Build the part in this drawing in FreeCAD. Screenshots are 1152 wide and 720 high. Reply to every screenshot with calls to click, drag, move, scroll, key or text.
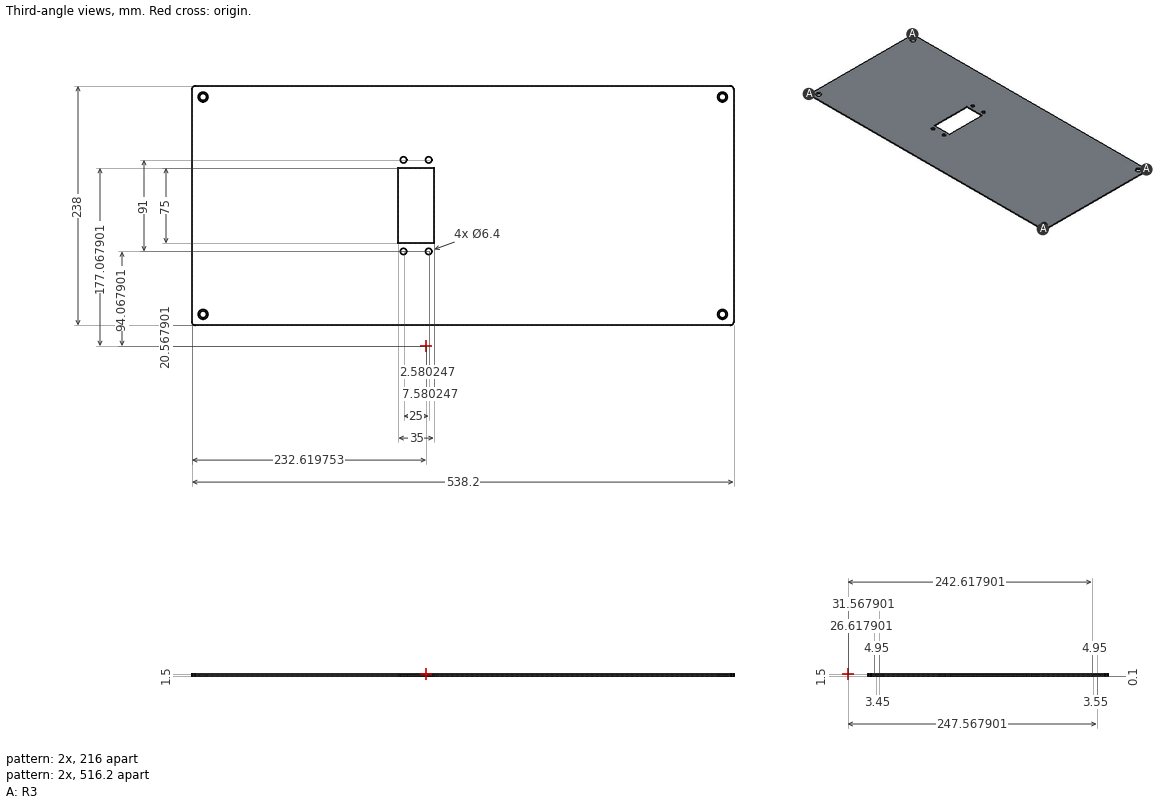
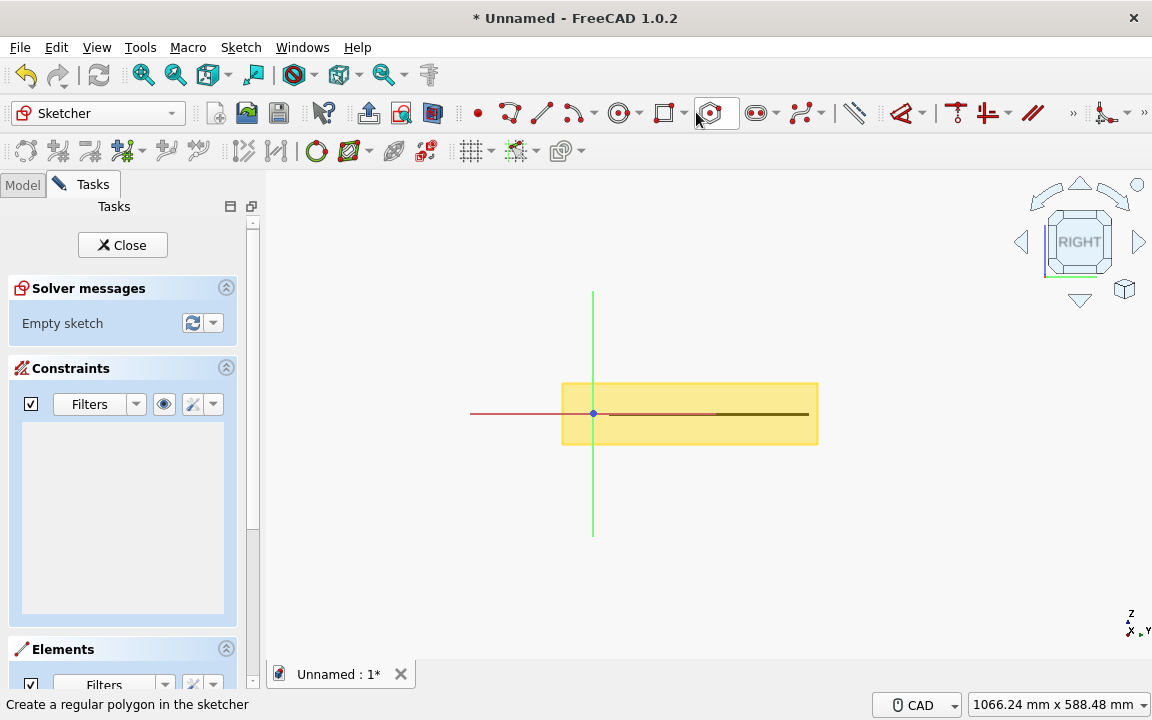
scroll(616, 414, up, 15)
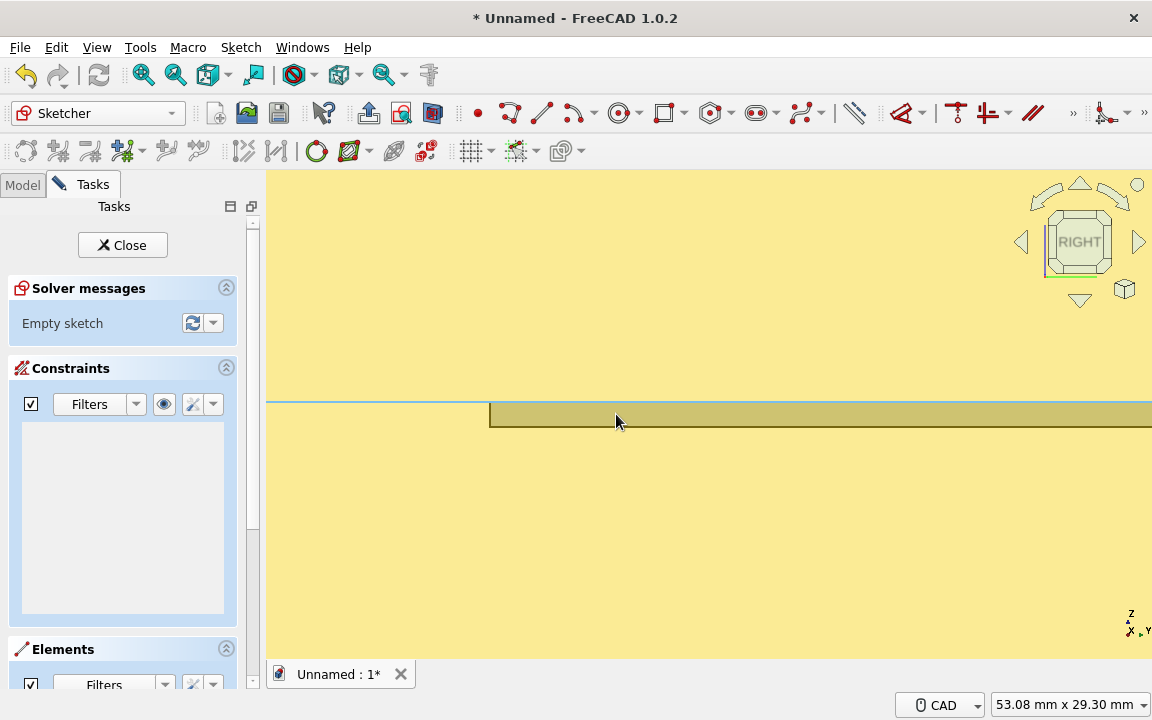
scroll(631, 407, up, 9)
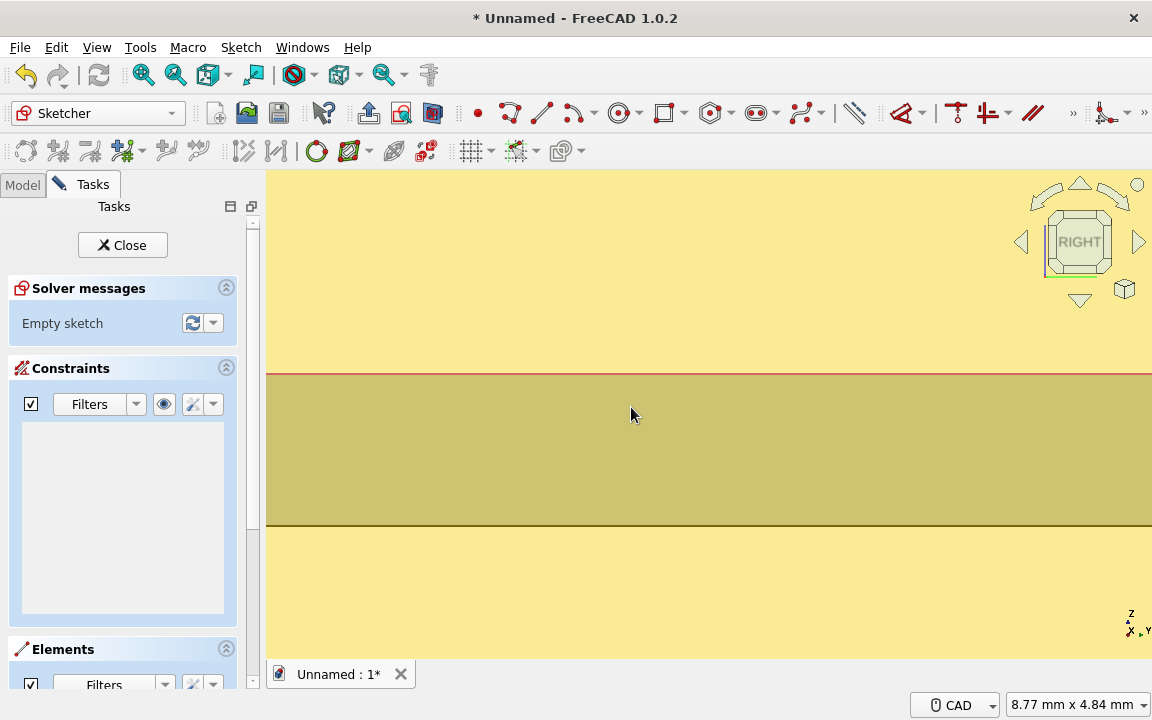
click(510, 114)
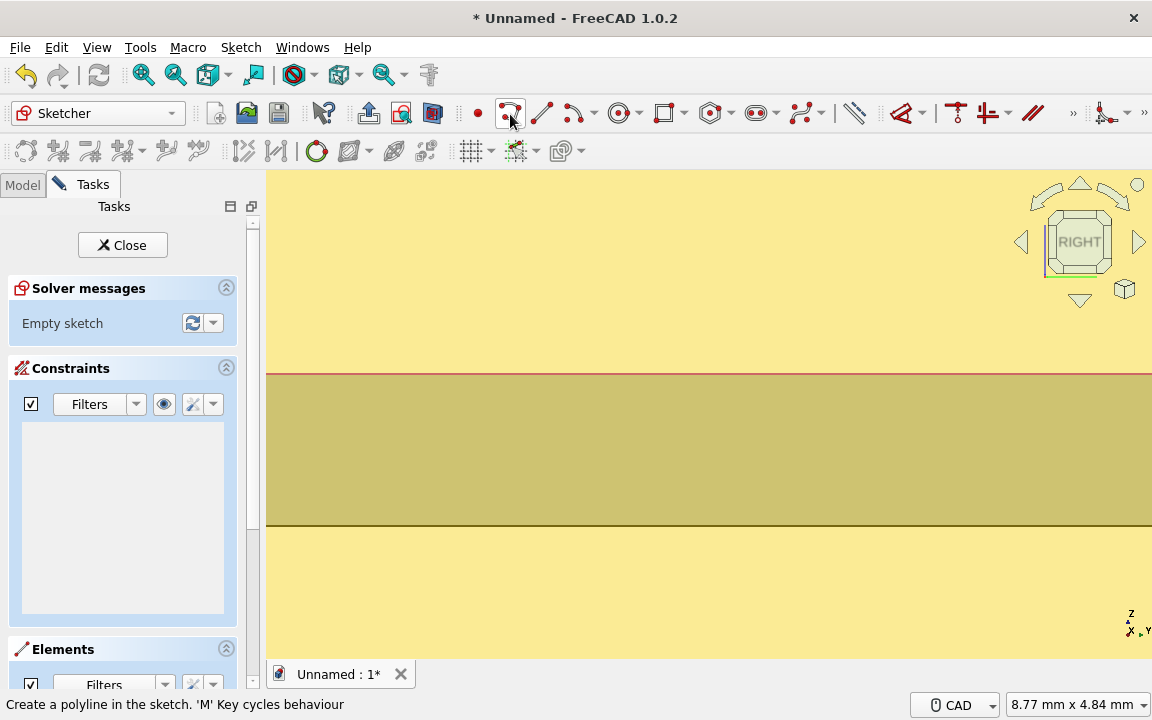
click(388, 374)
click(540, 526)
click(888, 526)
click(888, 383)
click(388, 374)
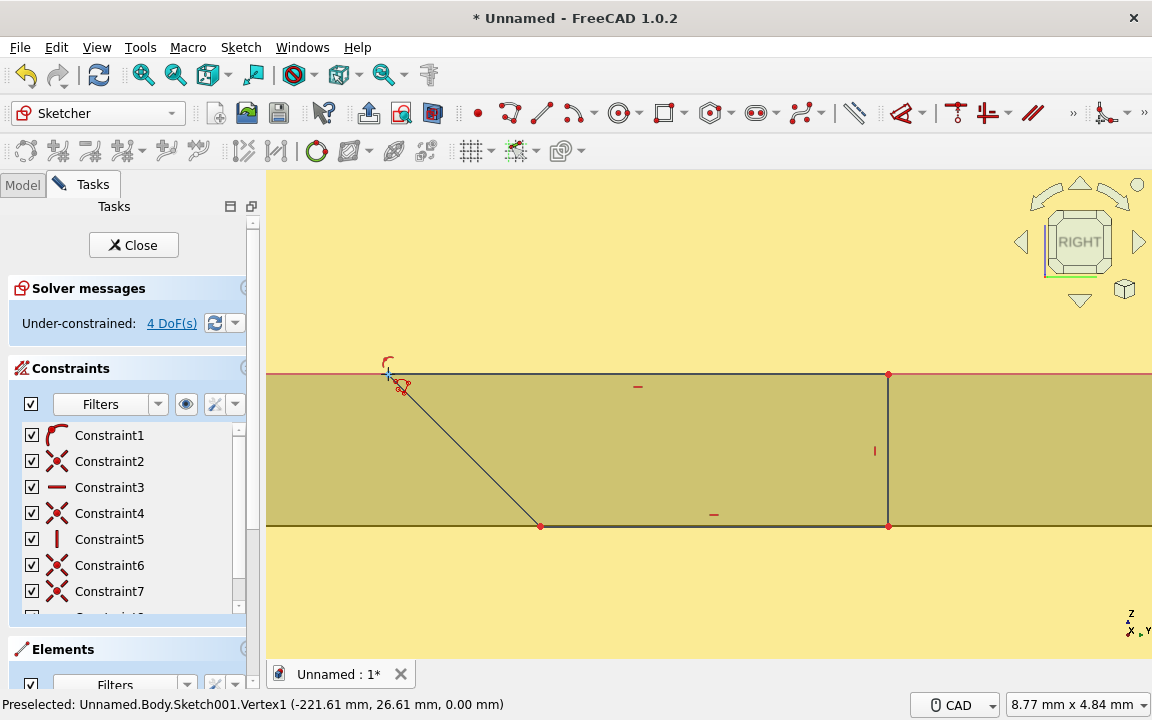
click(542, 114)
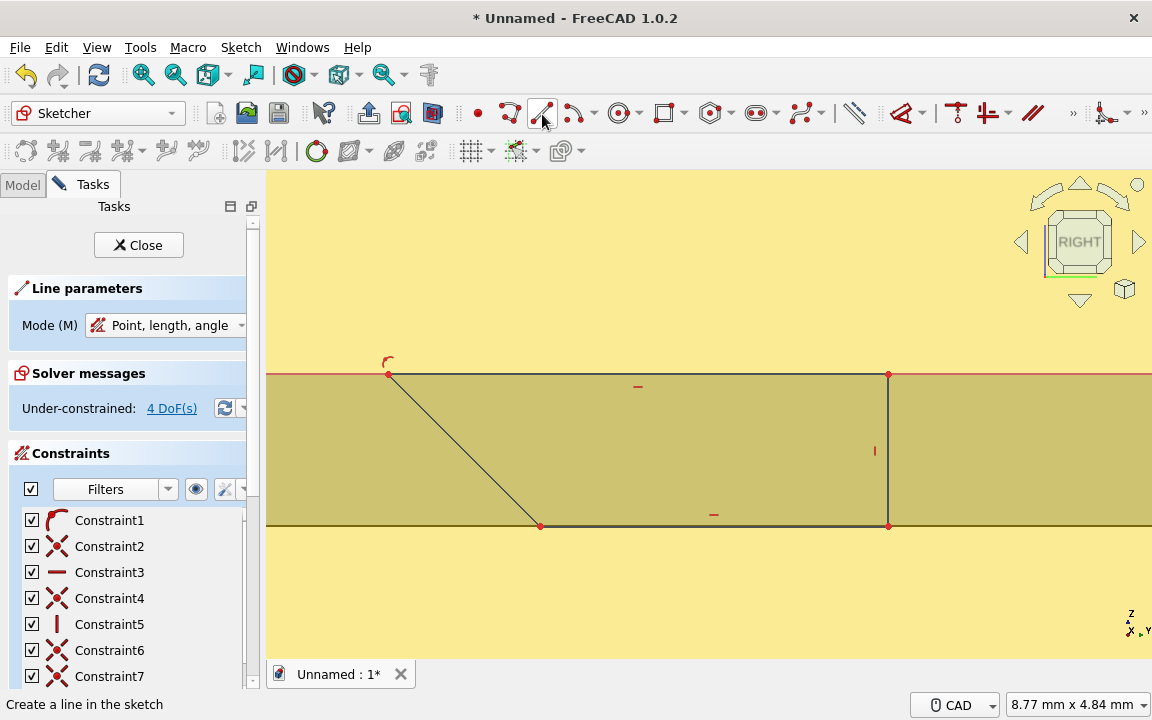
click(888, 354)
click(888, 294)
key(Escape)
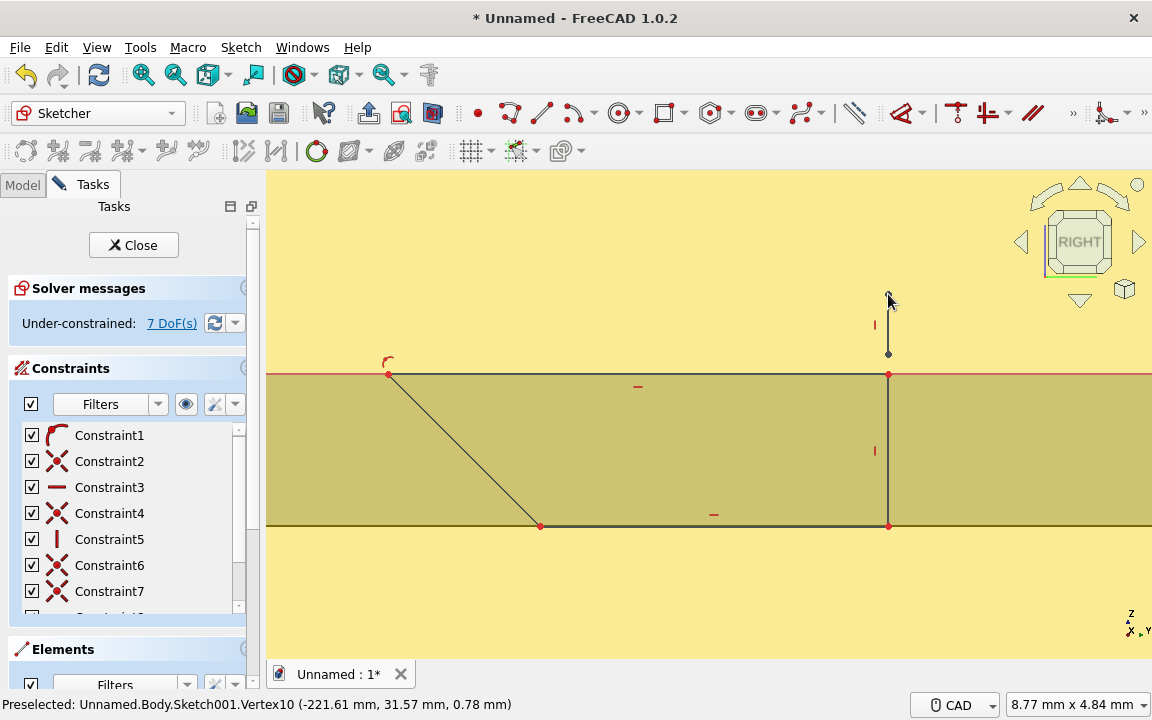
click(888, 337)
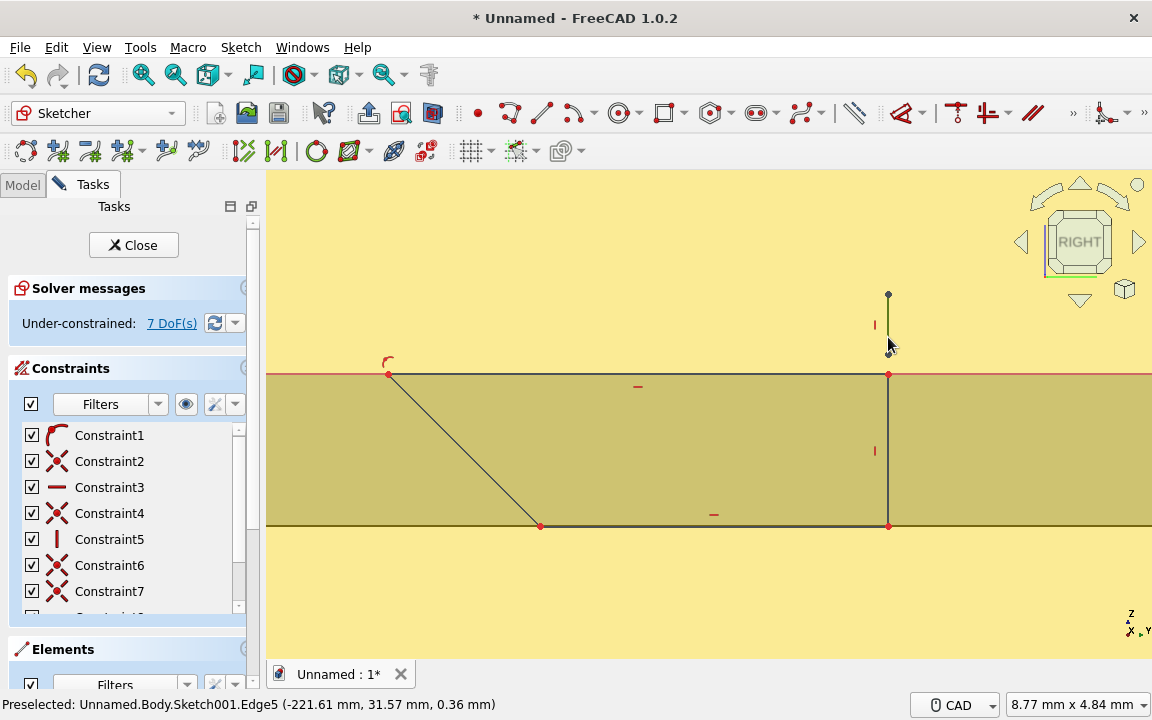
click(856, 114)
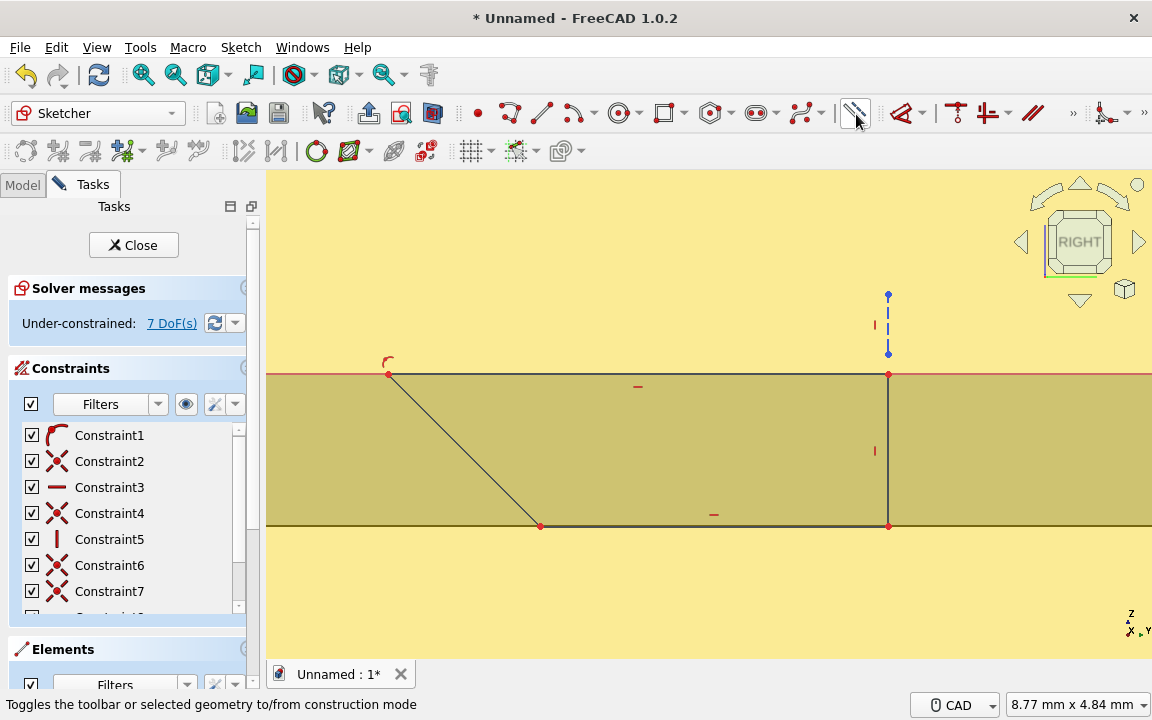
click(902, 114)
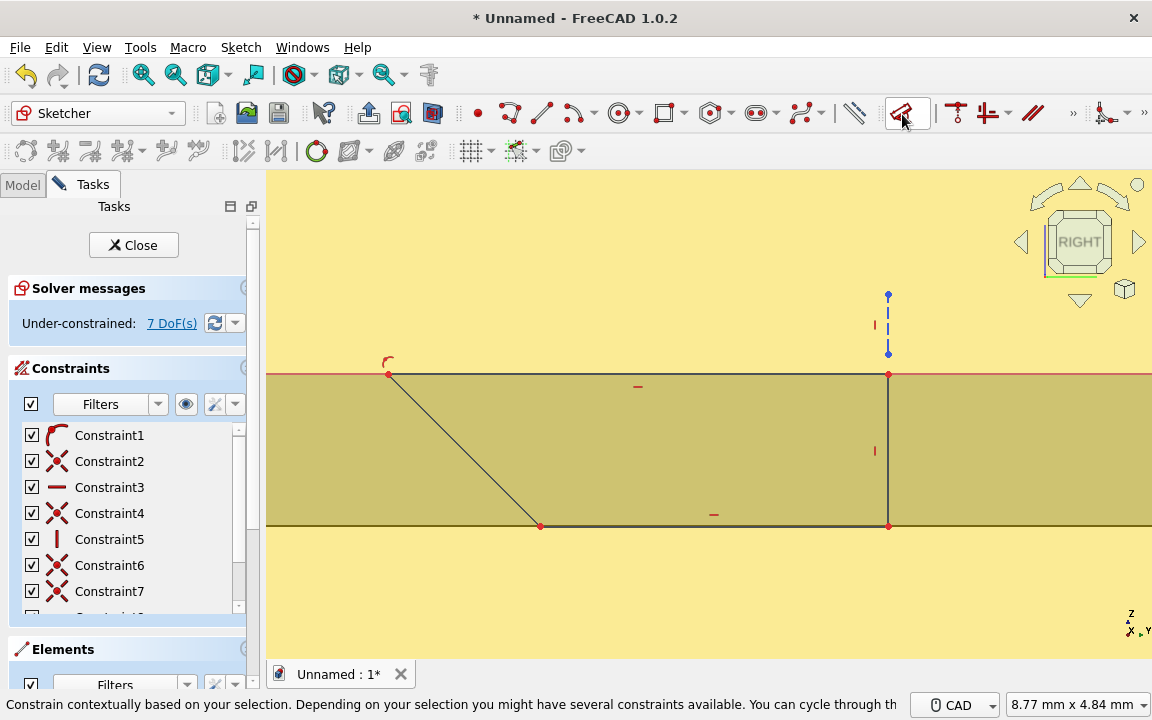
click(888, 481)
click(922, 451)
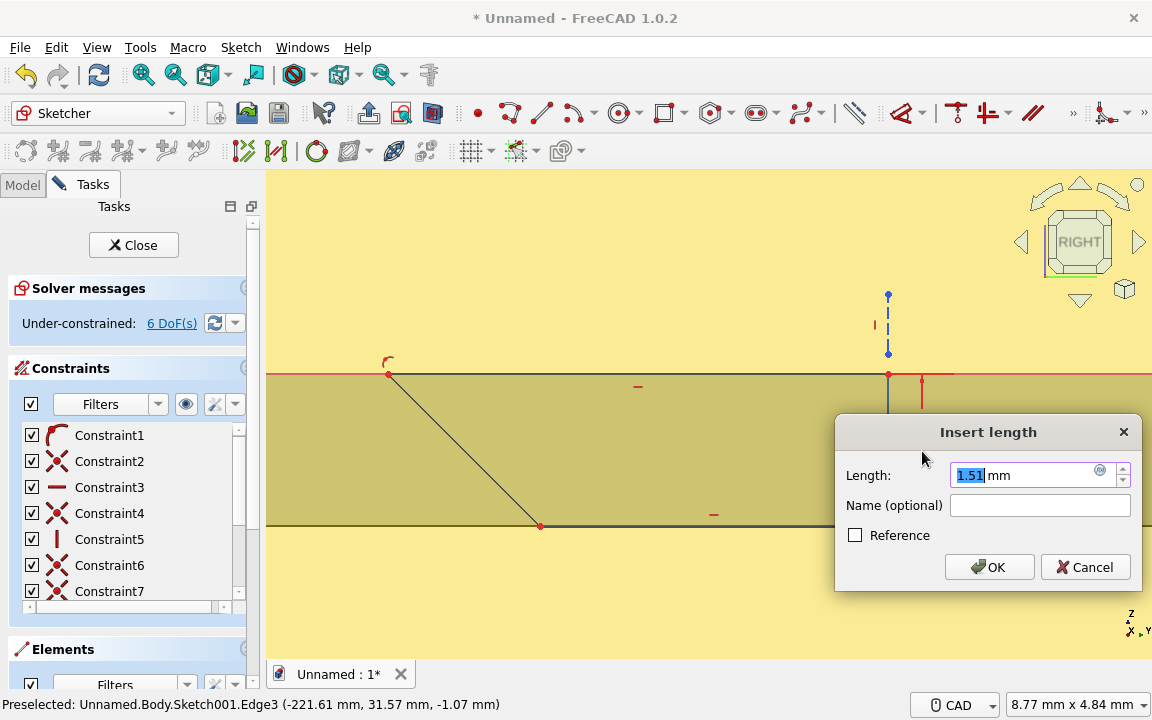
text(1.5)
key(Return)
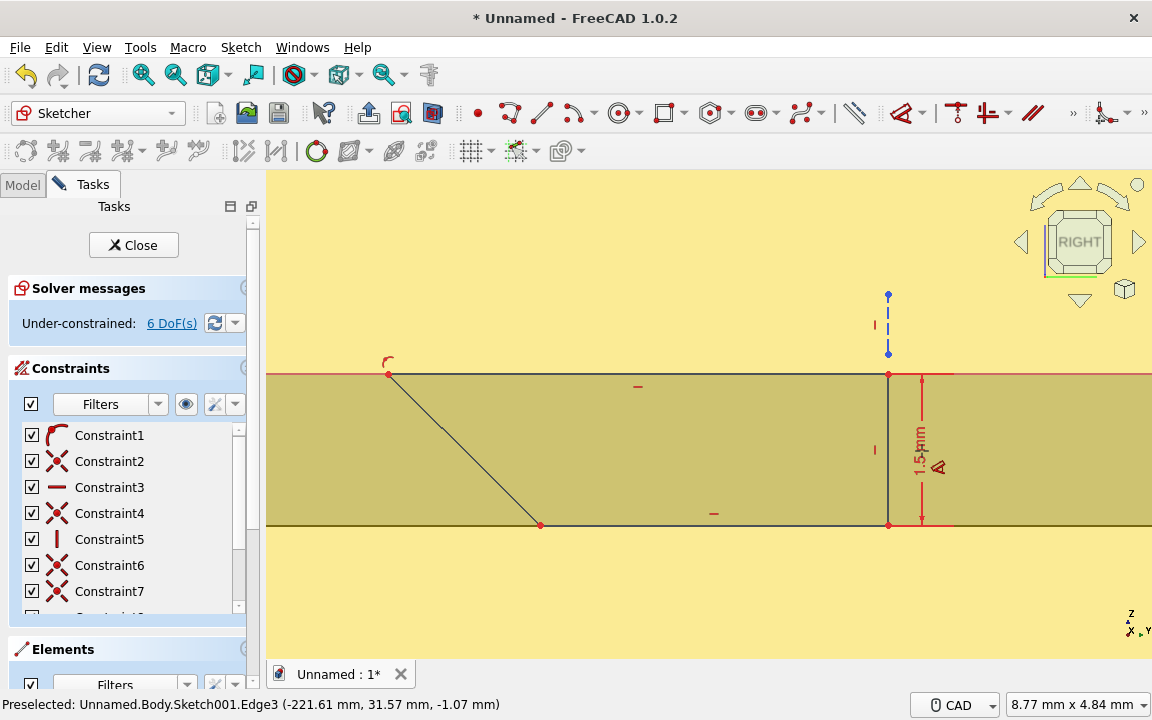
click(644, 526)
click(714, 560)